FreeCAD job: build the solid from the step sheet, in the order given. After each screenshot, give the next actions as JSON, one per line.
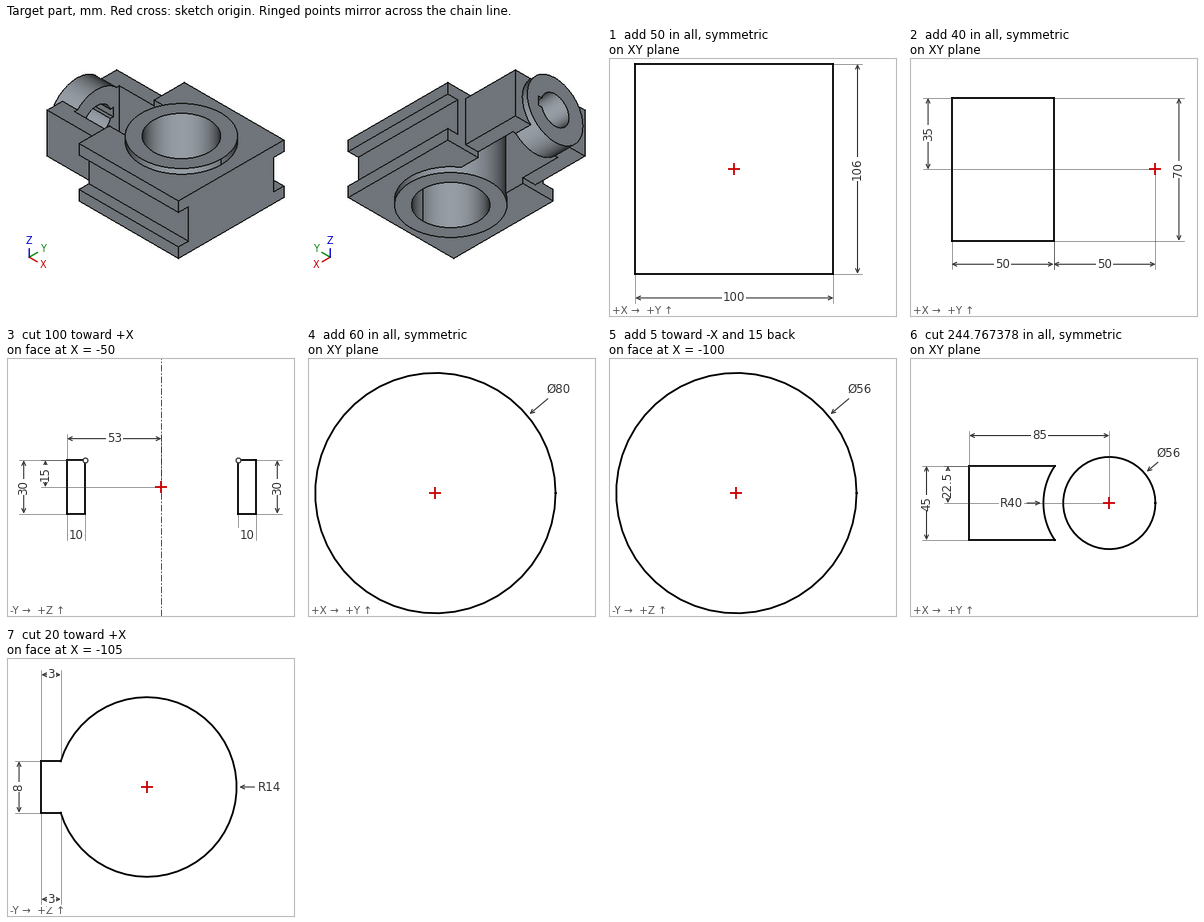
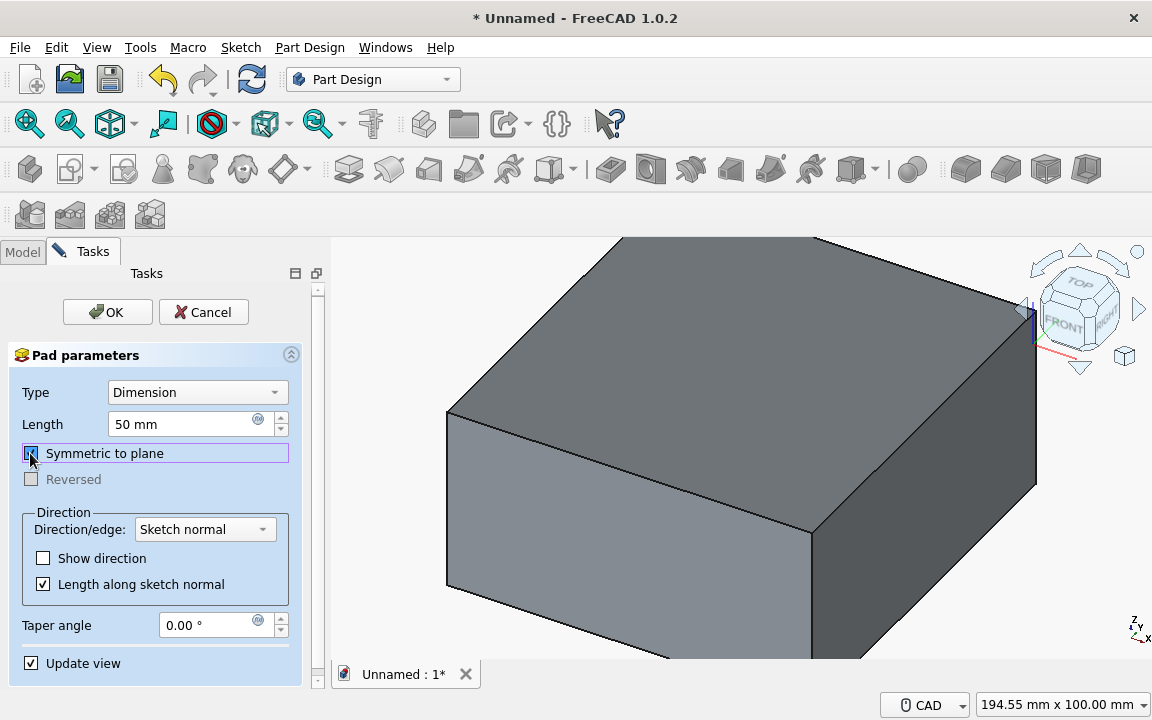
{"action": "left_click", "coordinate": [108, 312]}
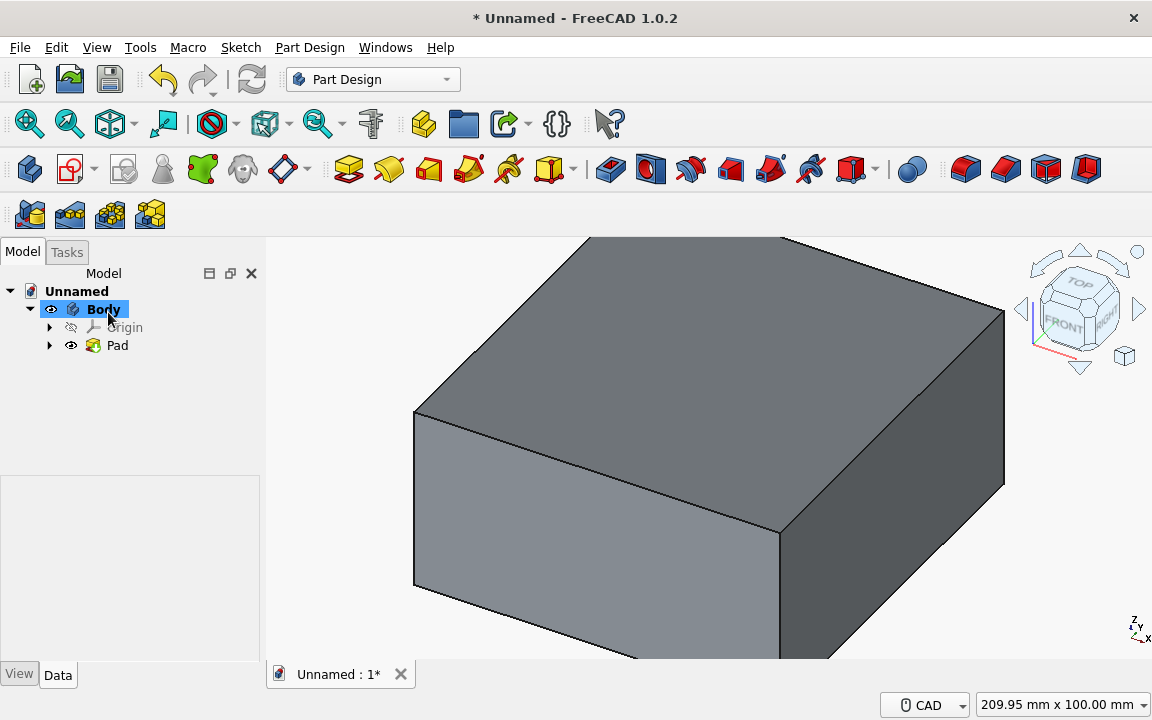
{"action": "left_click", "coordinate": [30, 124]}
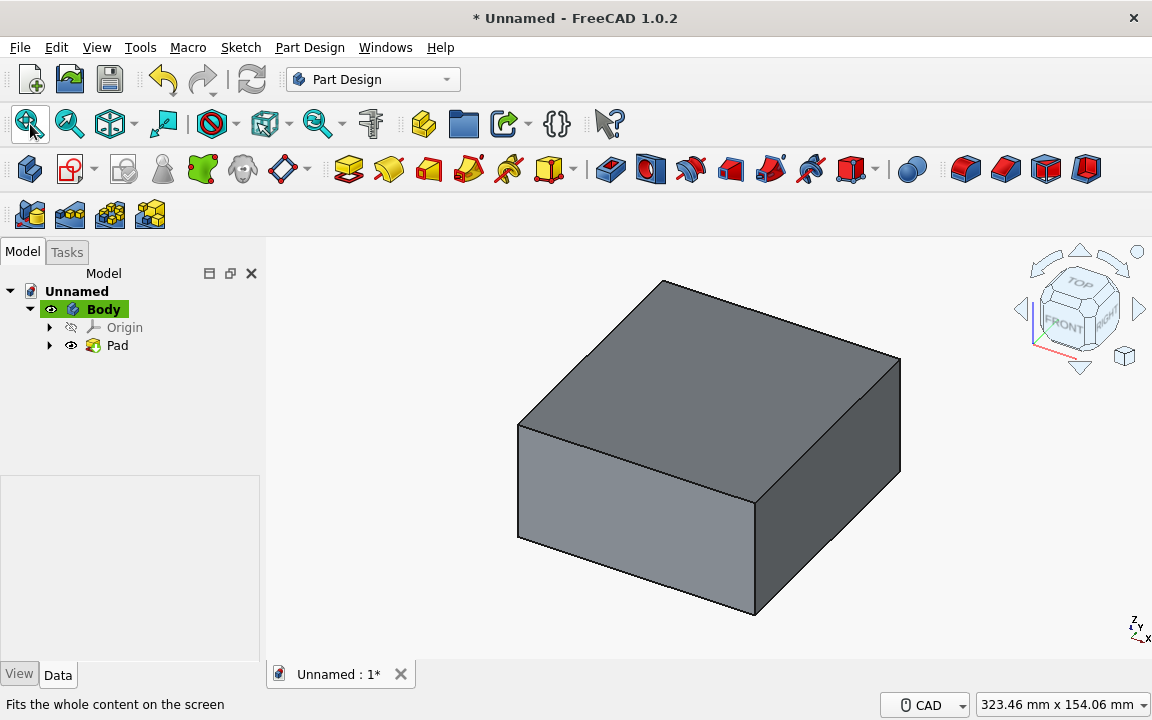
{"action": "left_click", "coordinate": [70, 170]}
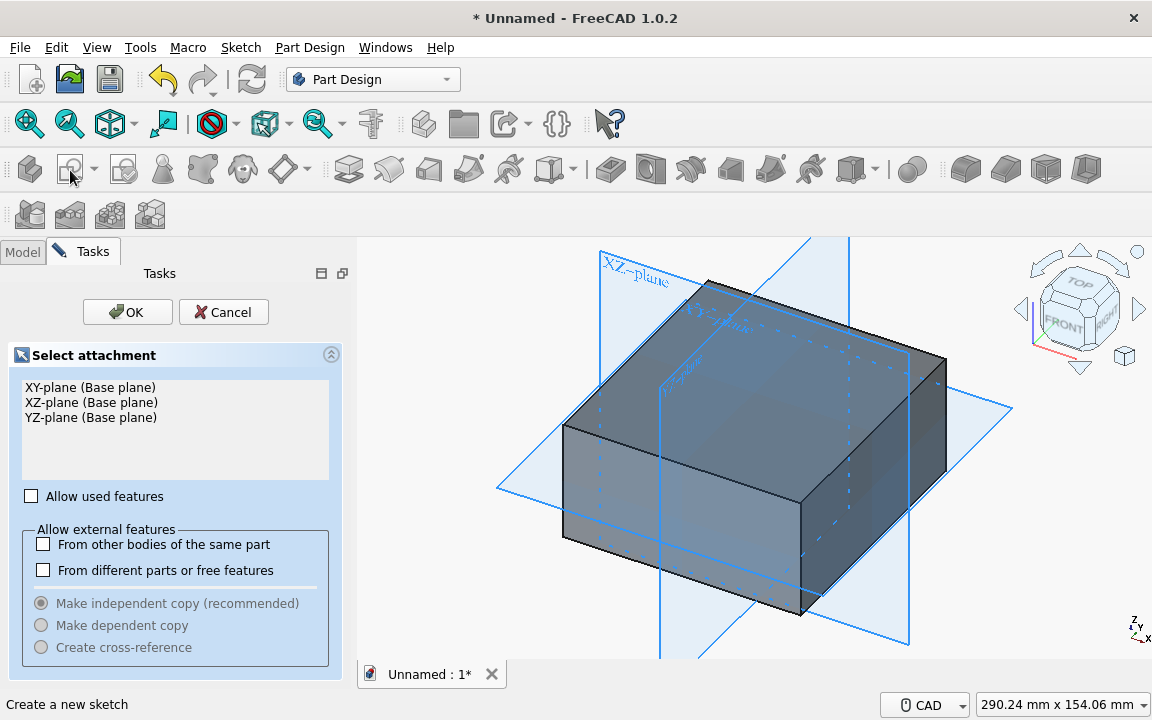
{"action": "left_click", "coordinate": [82, 388]}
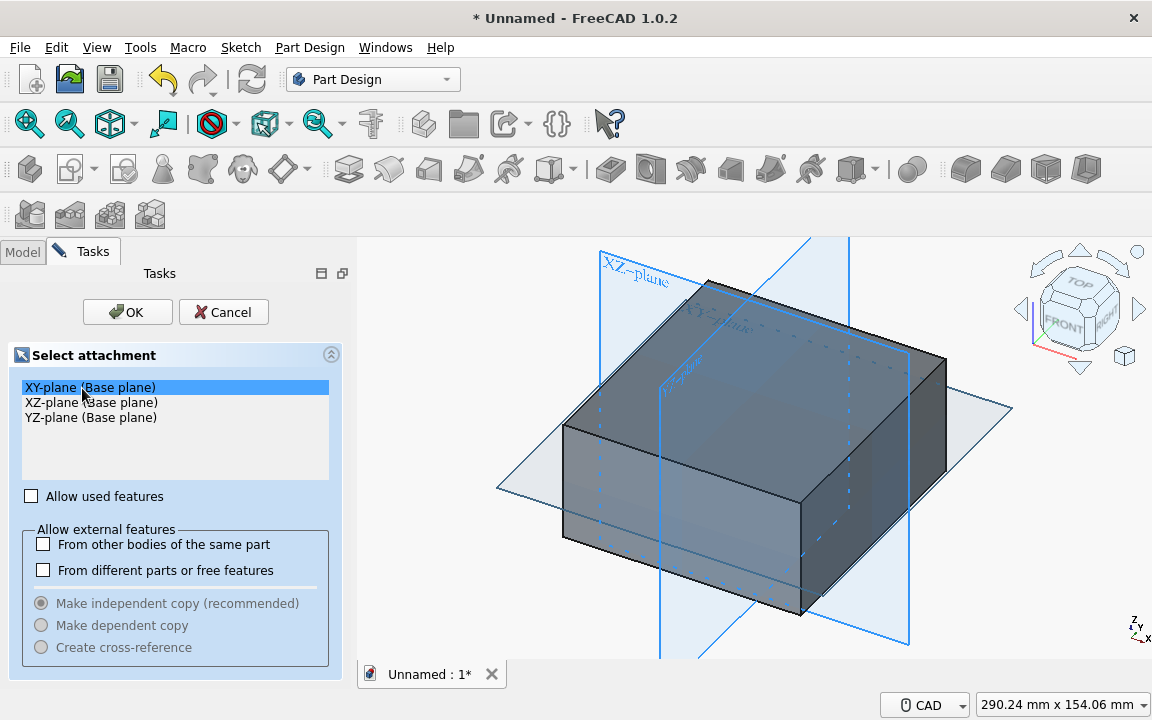
{"action": "left_click", "coordinate": [128, 312]}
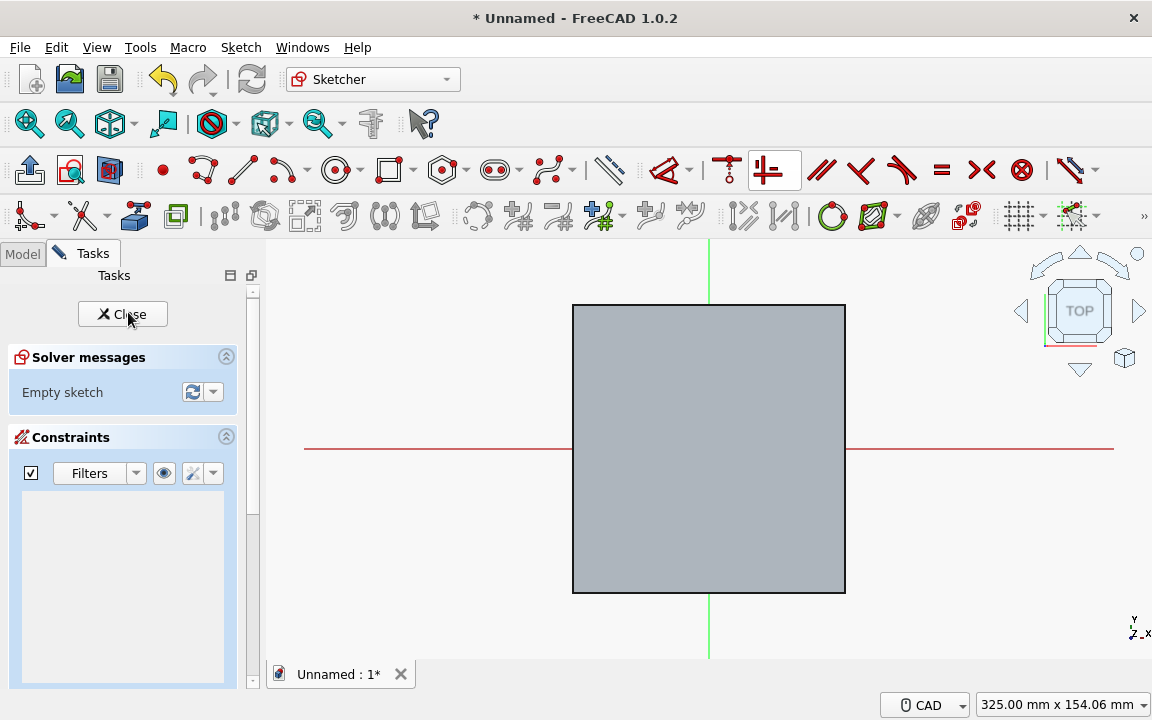
{"action": "left_click", "coordinate": [110, 170]}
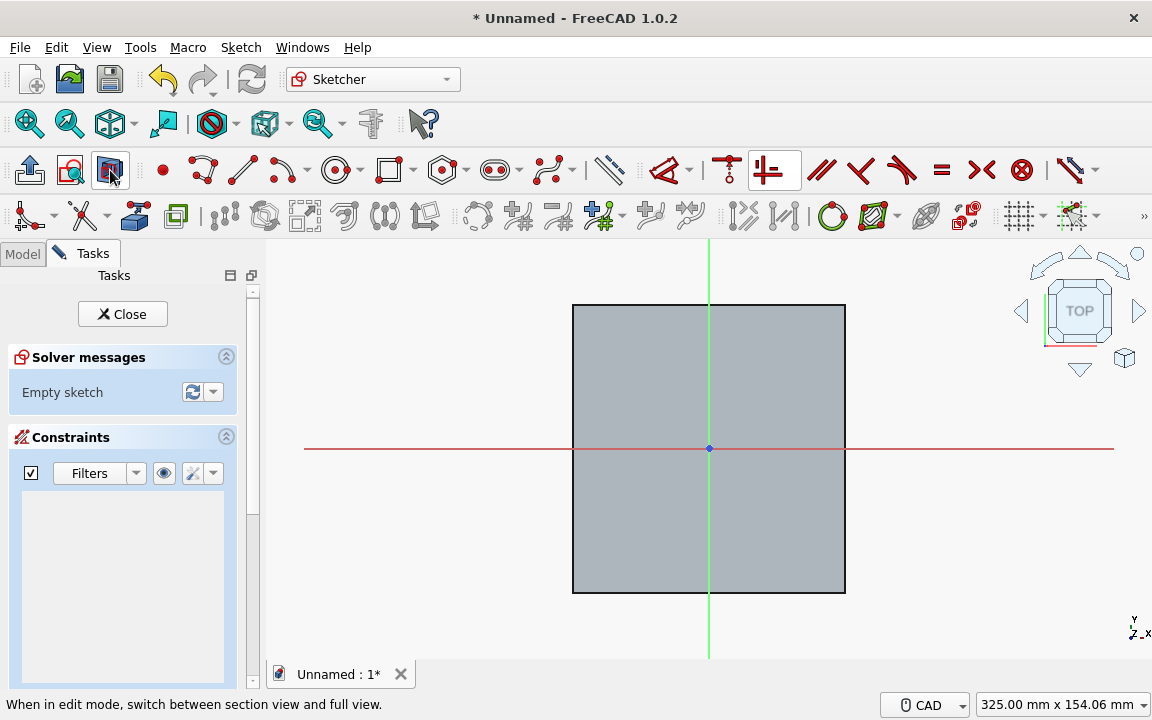
{"action": "left_click", "coordinate": [390, 170]}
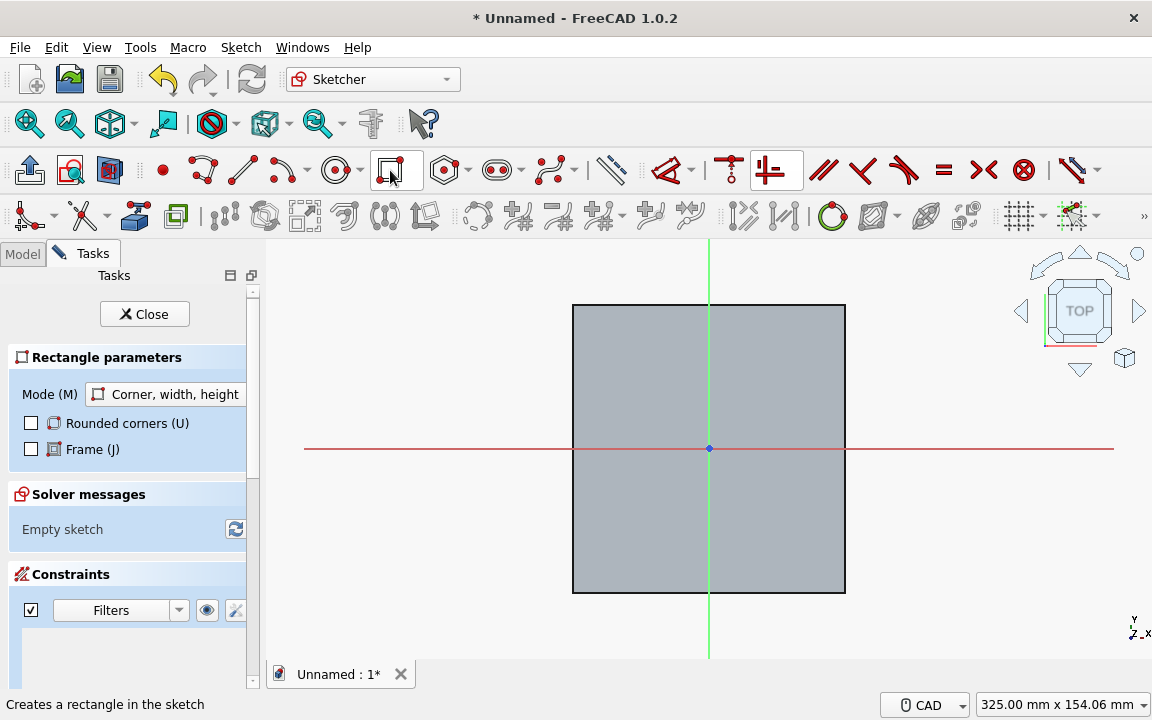
{"action": "left_click", "coordinate": [436, 354]}
{"action": "mouse_move", "coordinate": [573, 544]}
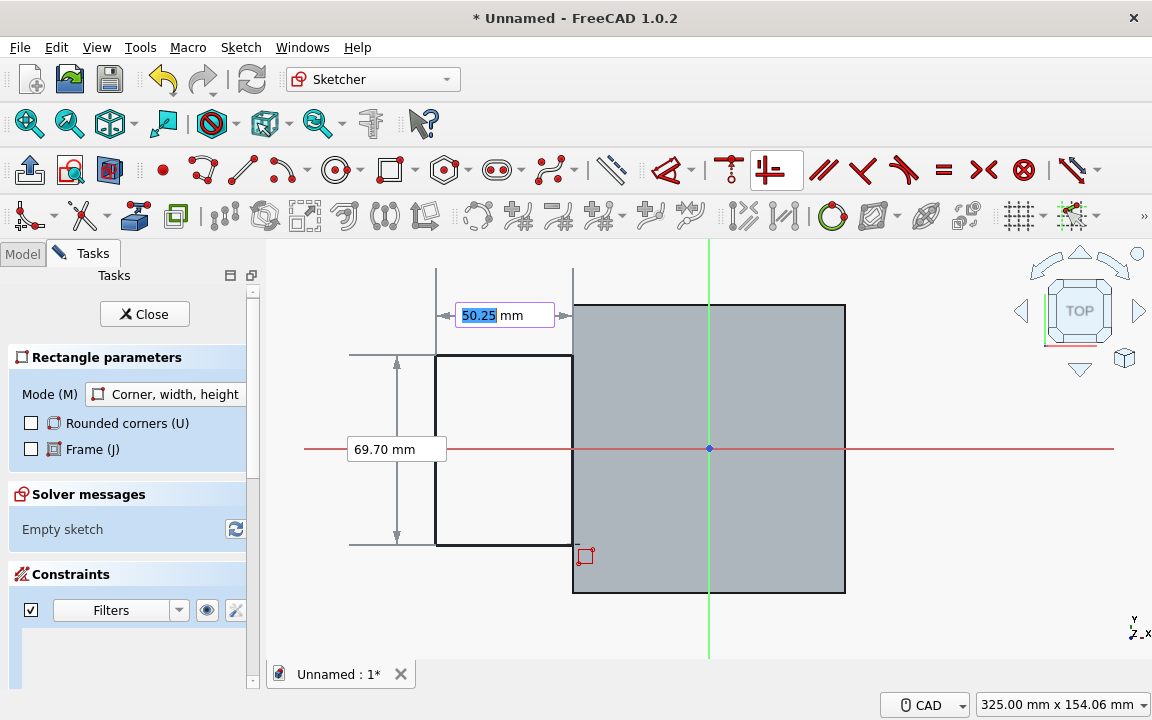
{"action": "type", "text": "50"}
{"action": "key", "text": "Tab"}
{"action": "type", "text": "70"}
{"action": "key", "text": "Return"}
{"action": "key", "text": "Escape"}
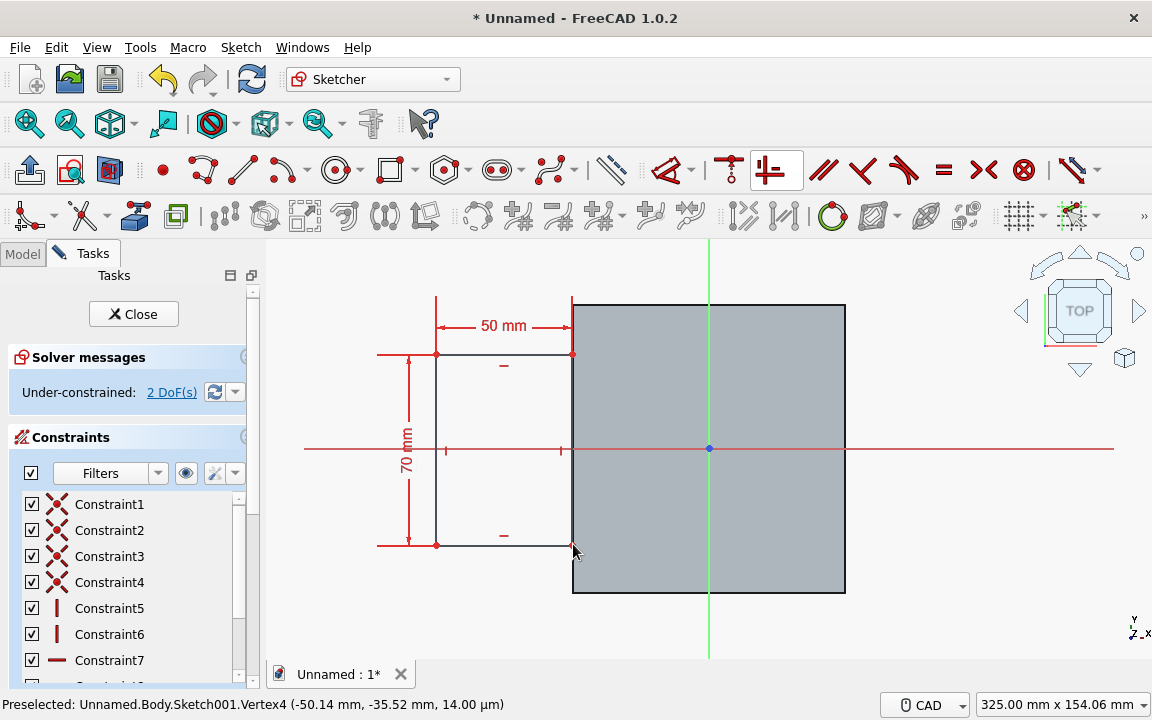
{"action": "left_click", "coordinate": [666, 170]}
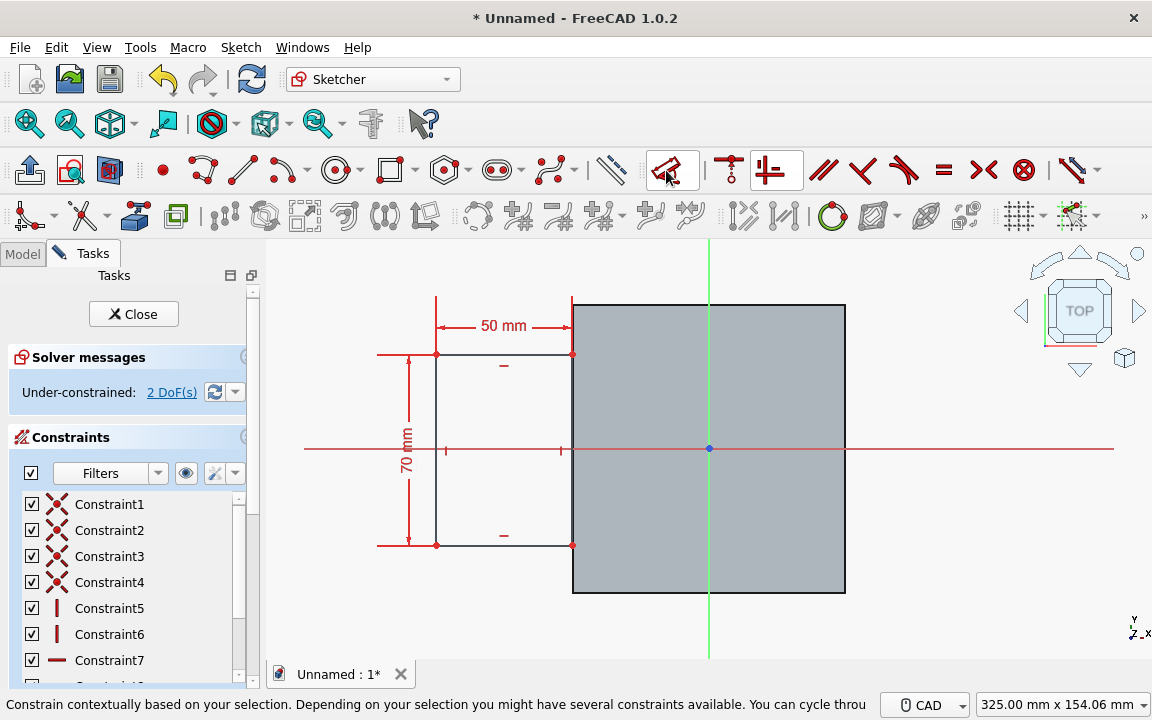
{"action": "left_click", "coordinate": [436, 355]}
{"action": "left_click", "coordinate": [402, 402]}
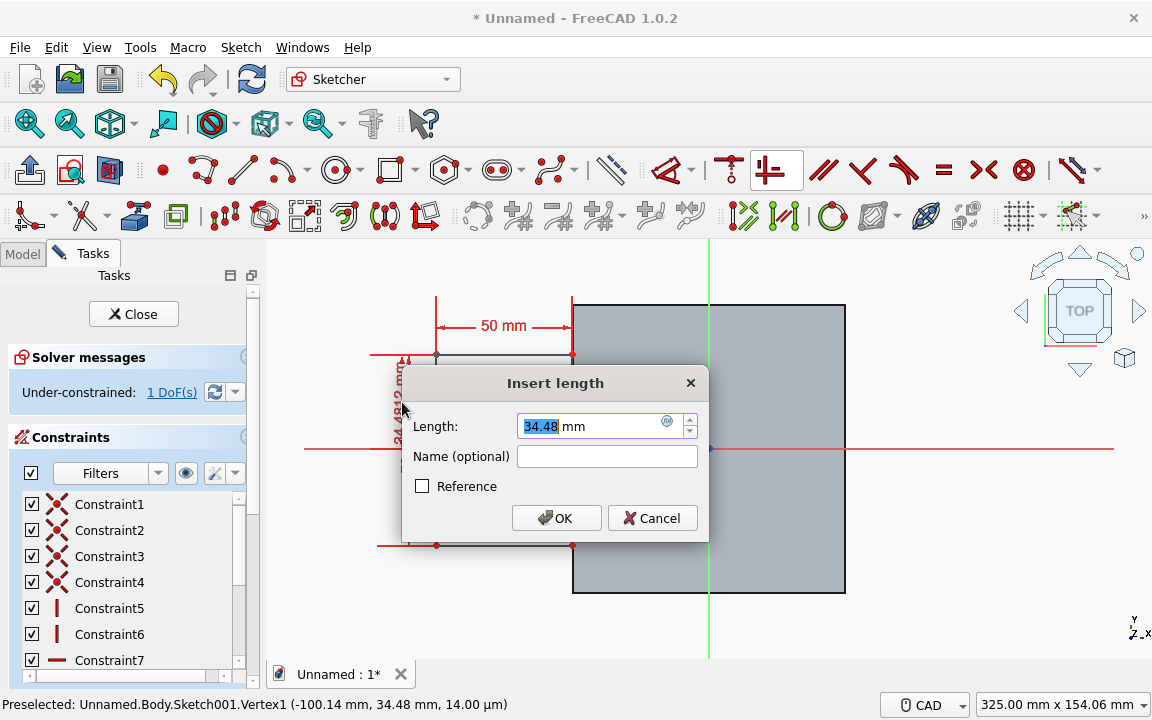
{"action": "type", "text": "35"}
{"action": "key", "text": "Return"}